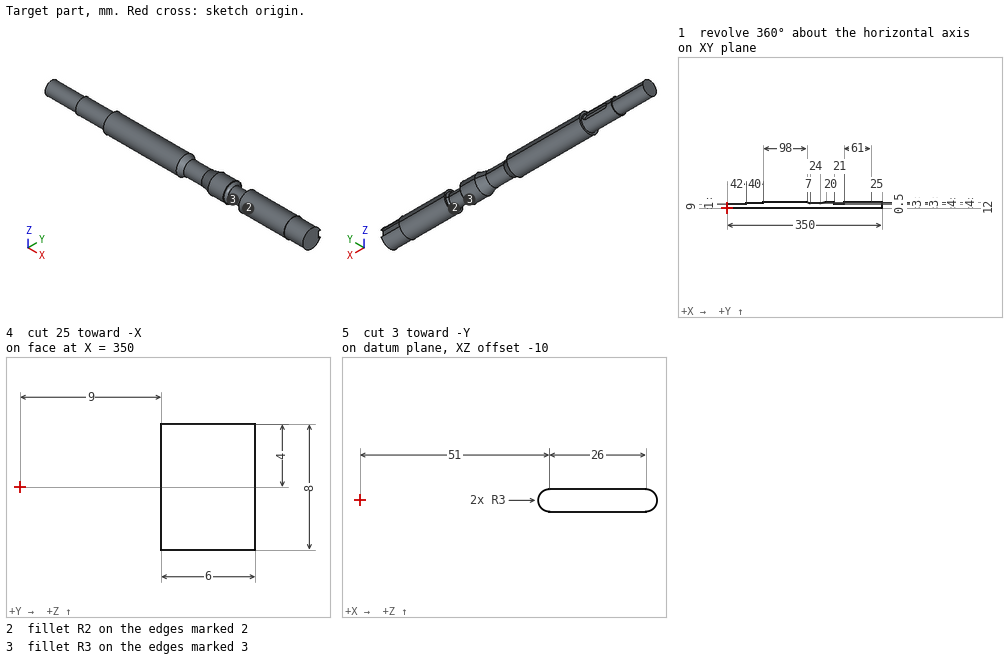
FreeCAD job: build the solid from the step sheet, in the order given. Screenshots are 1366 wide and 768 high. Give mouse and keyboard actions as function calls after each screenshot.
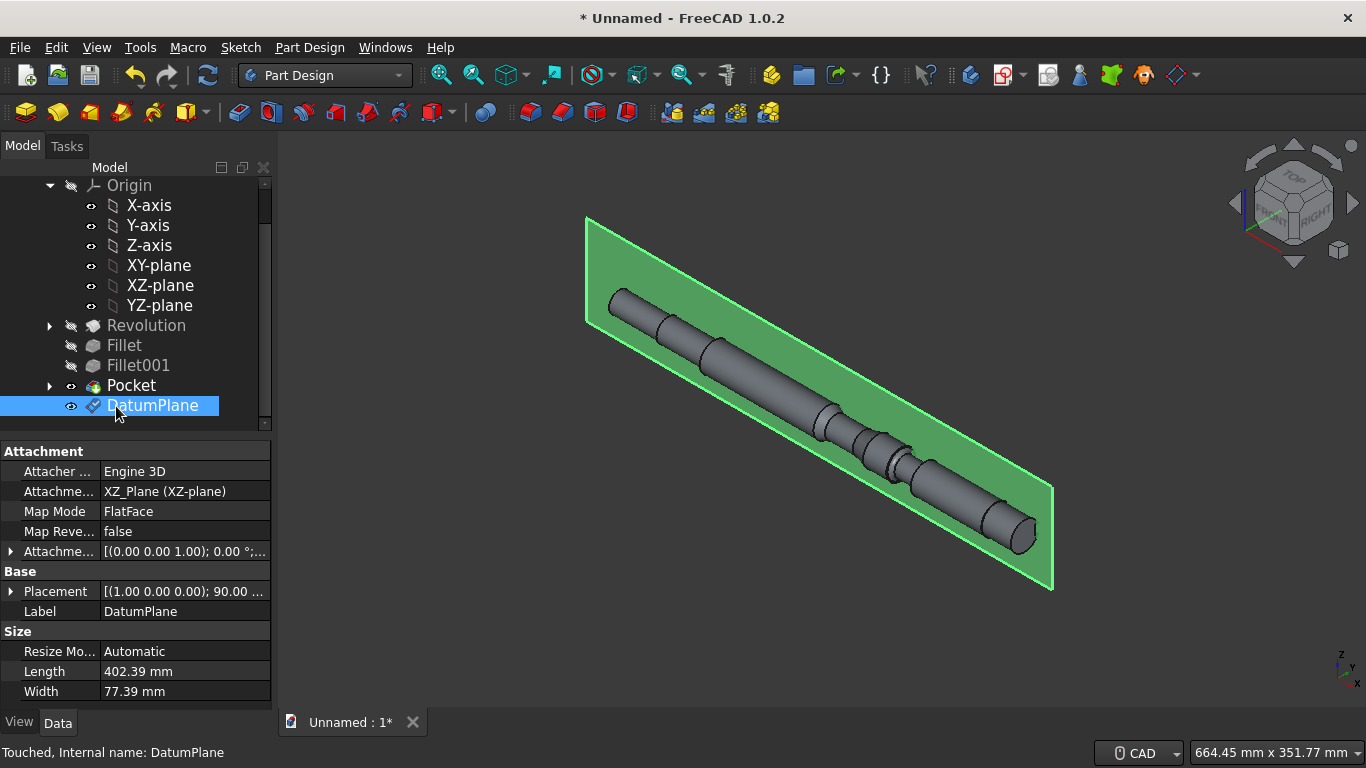
click(1004, 76)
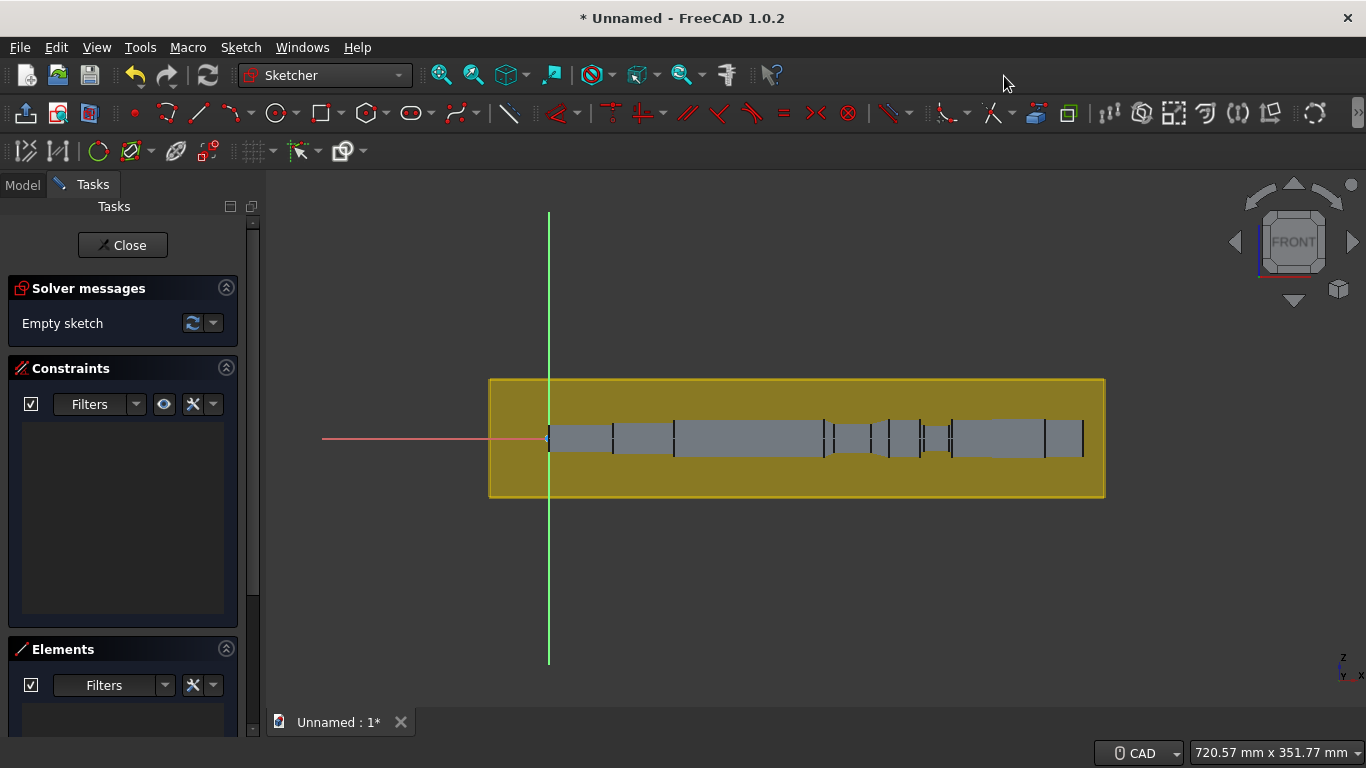
click(90, 114)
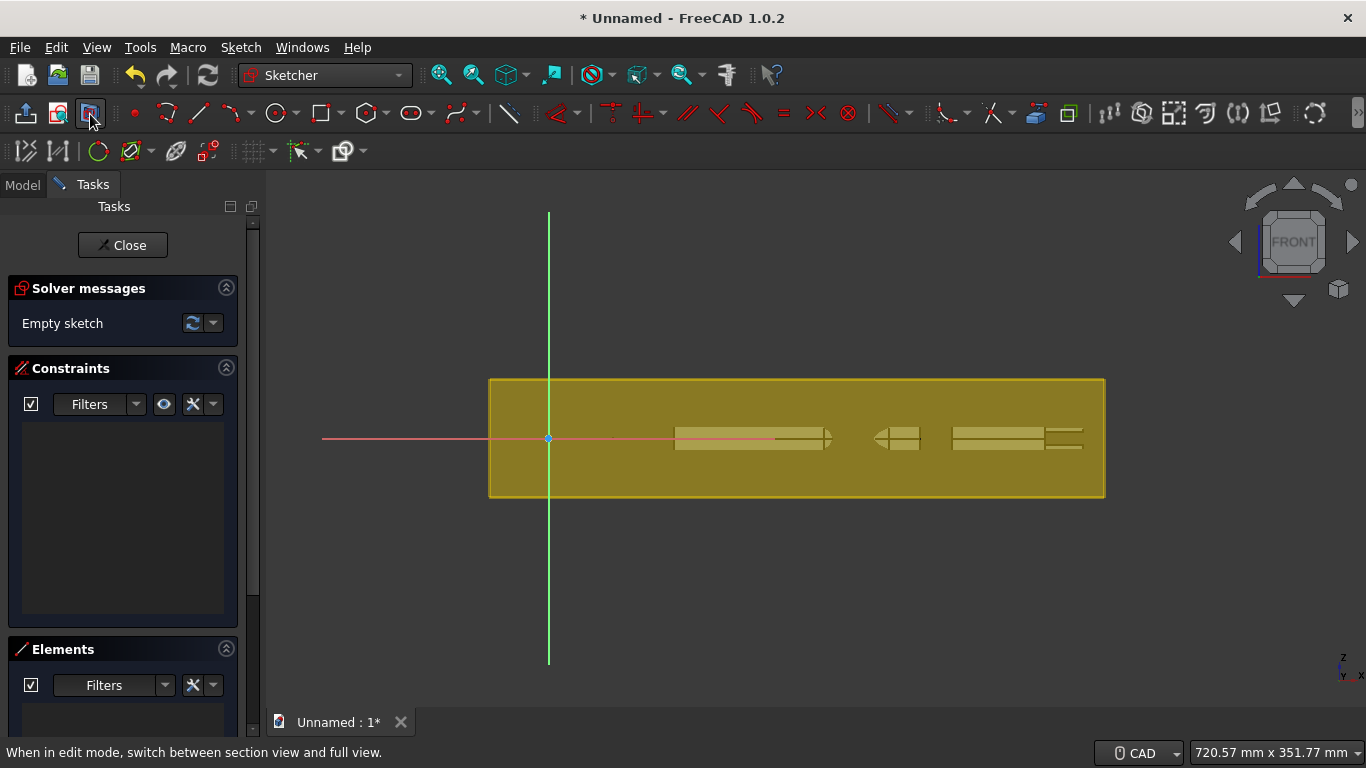
scroll(638, 438, up, 13)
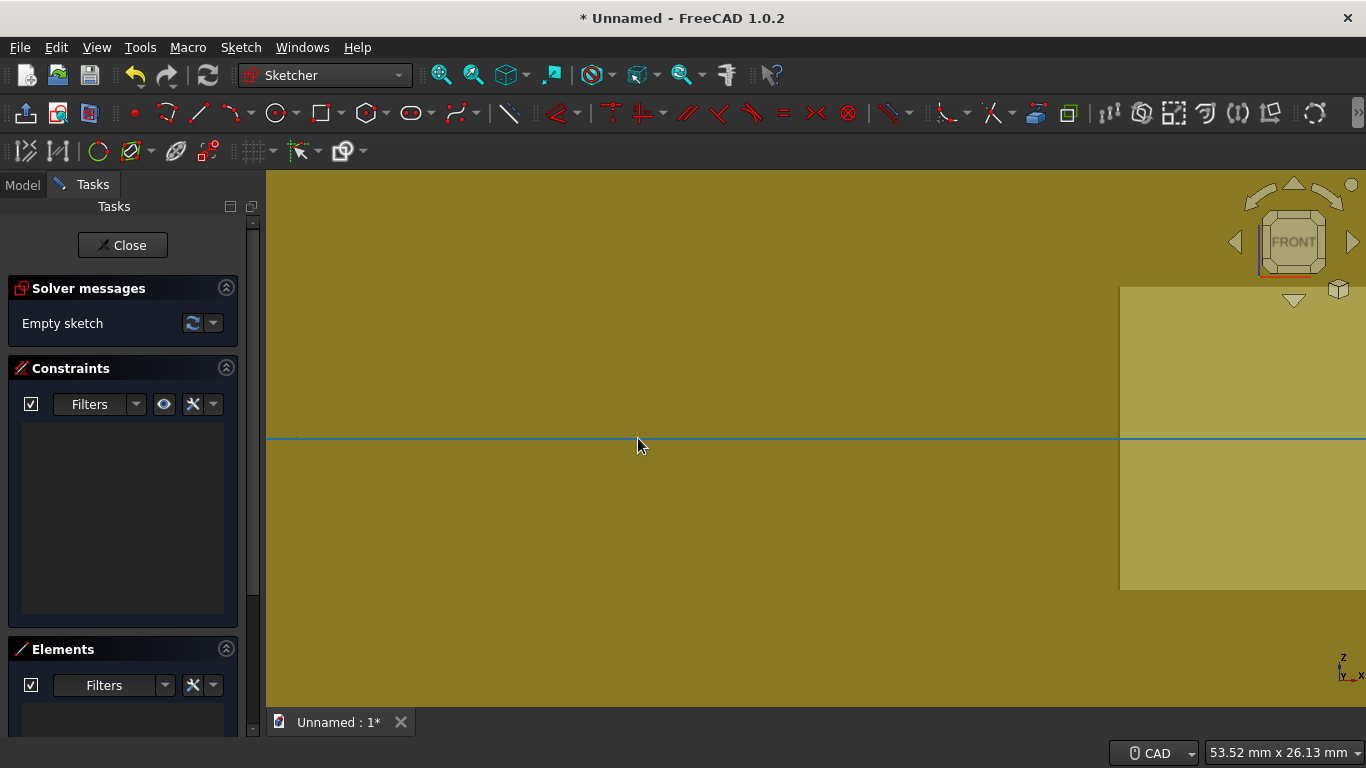
click(412, 114)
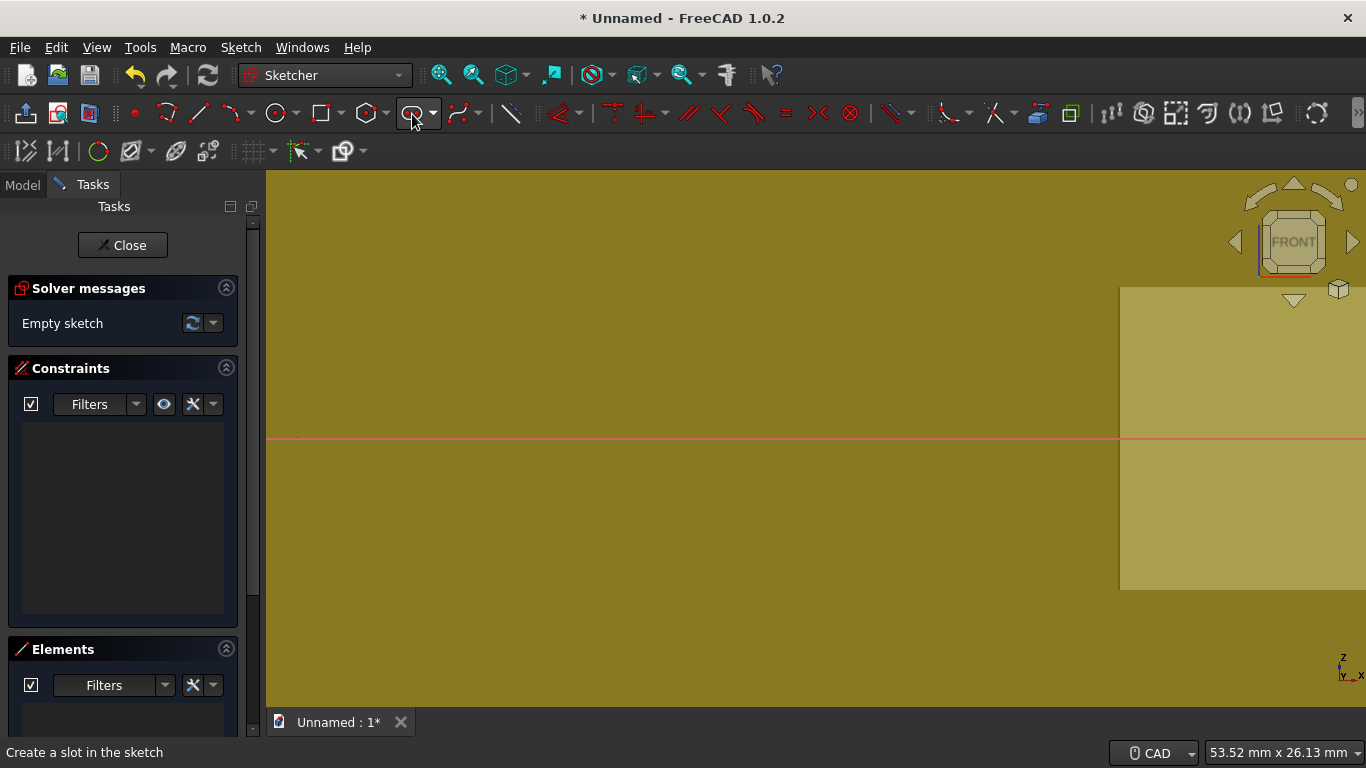
click(482, 439)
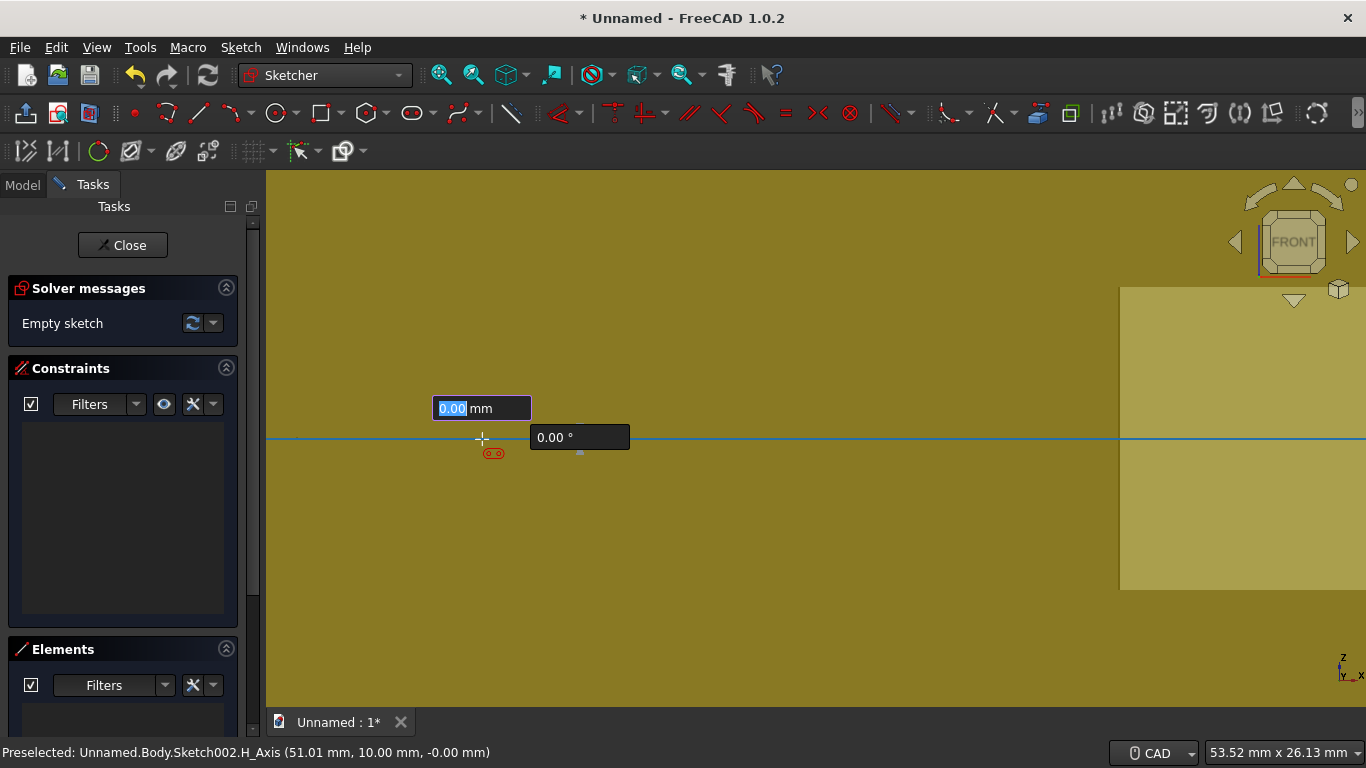
click(1016, 430)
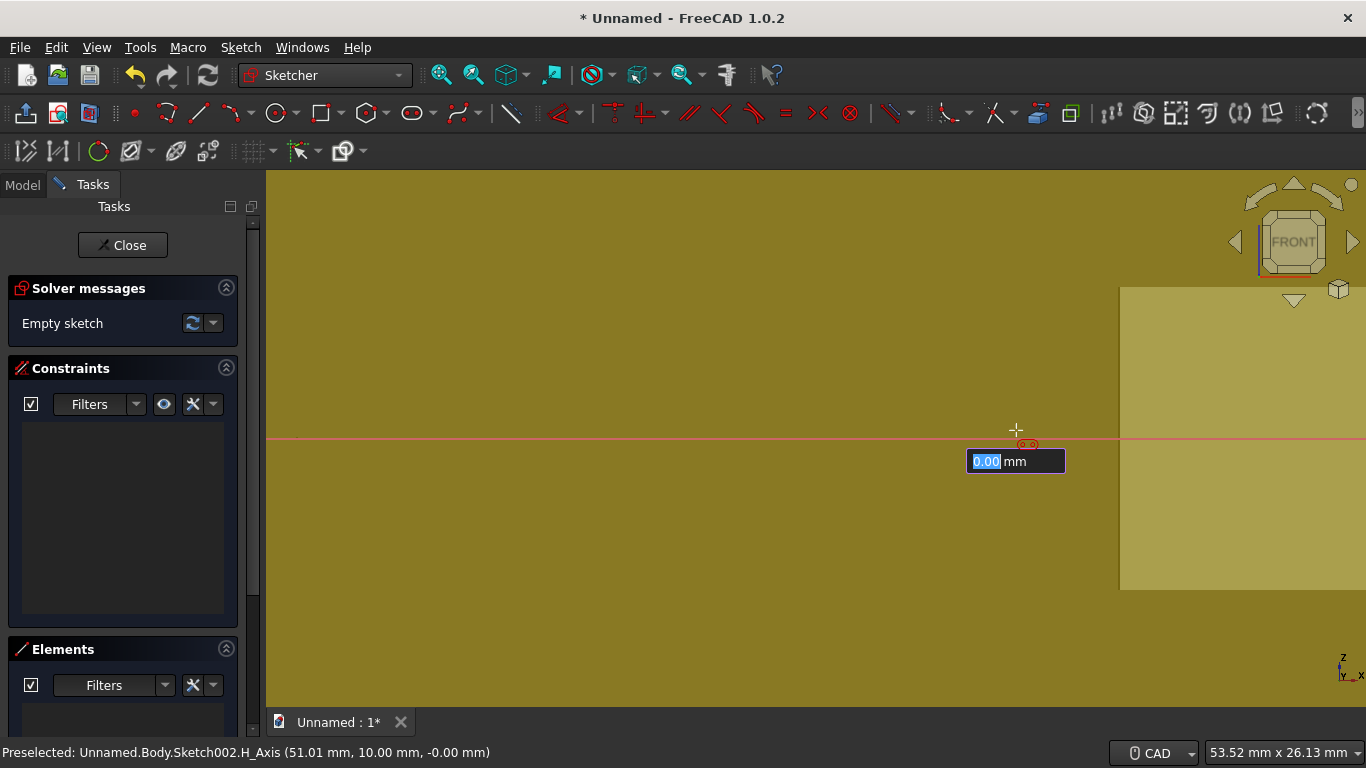
click(749, 500)
key(Escape)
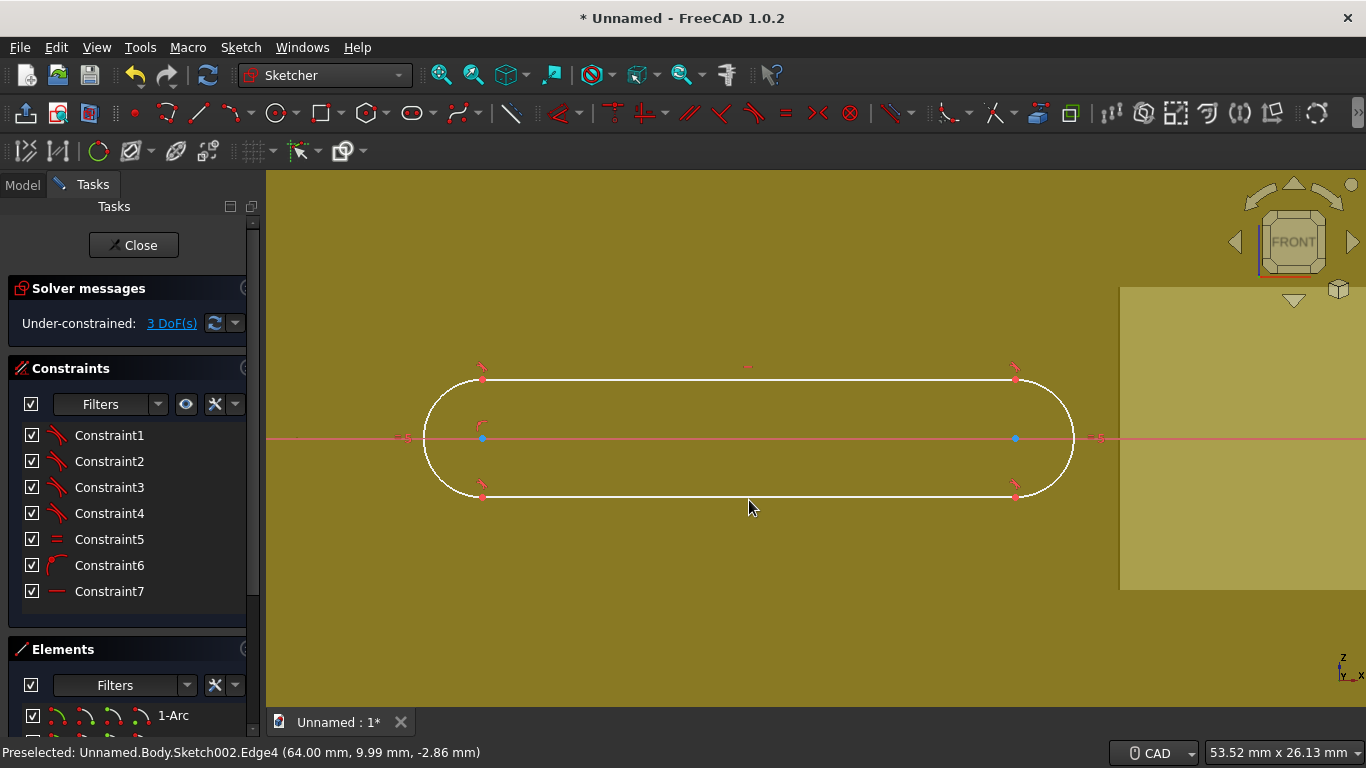
click(558, 114)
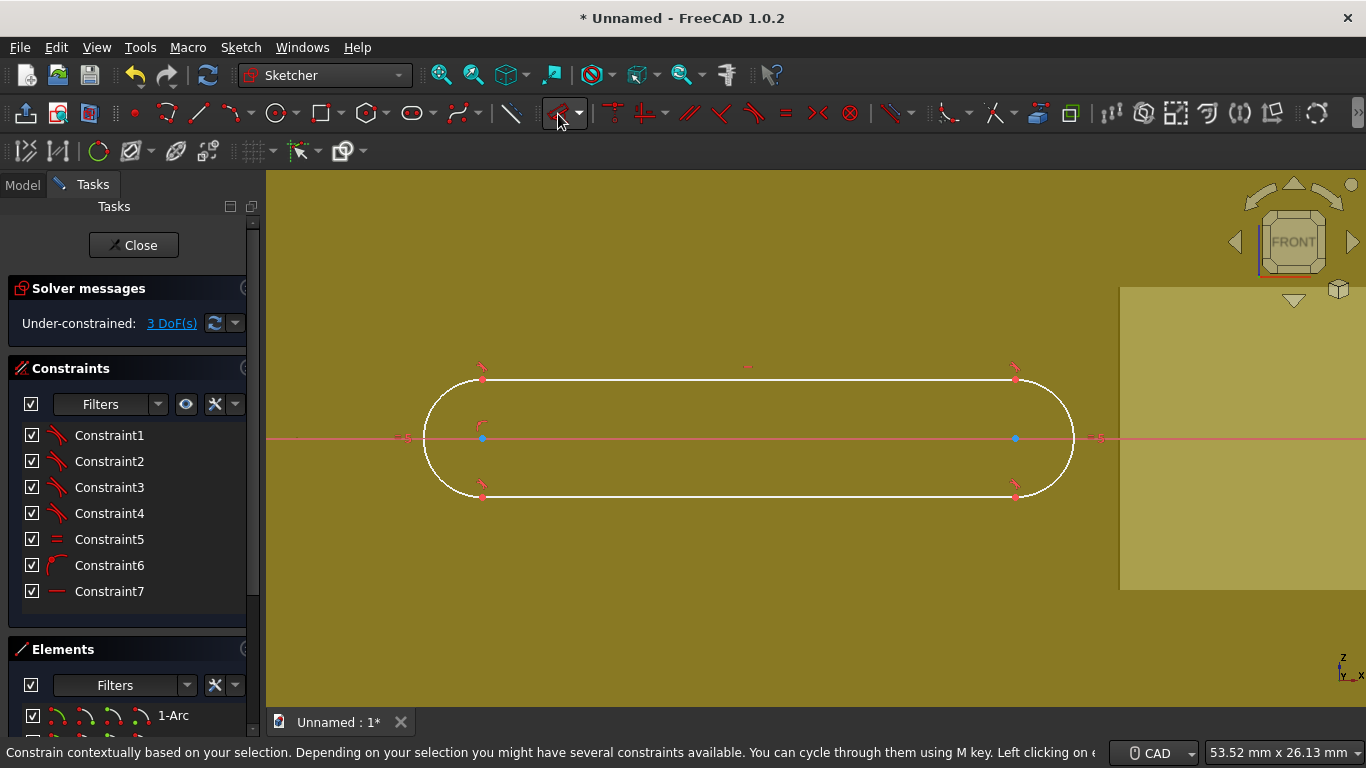
click(435, 404)
click(409, 385)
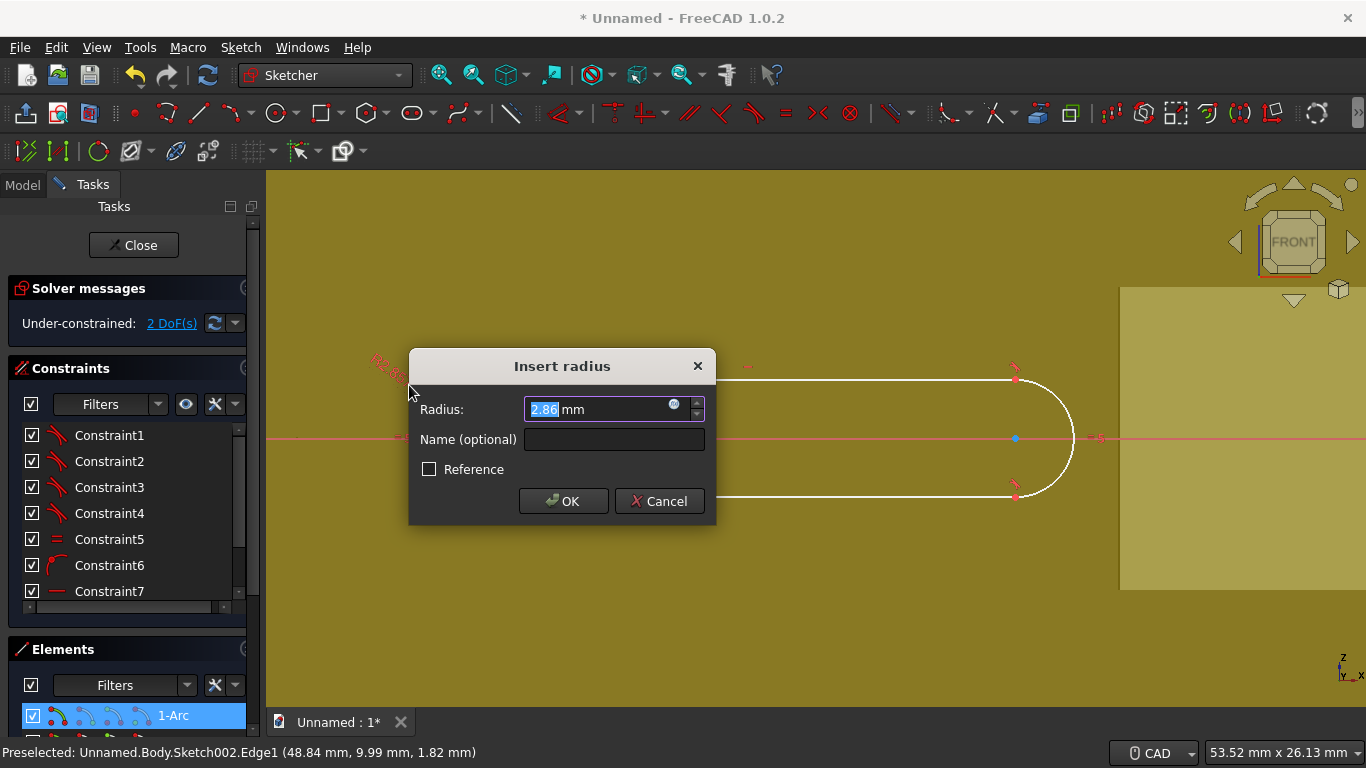
text(3)
key(Return)